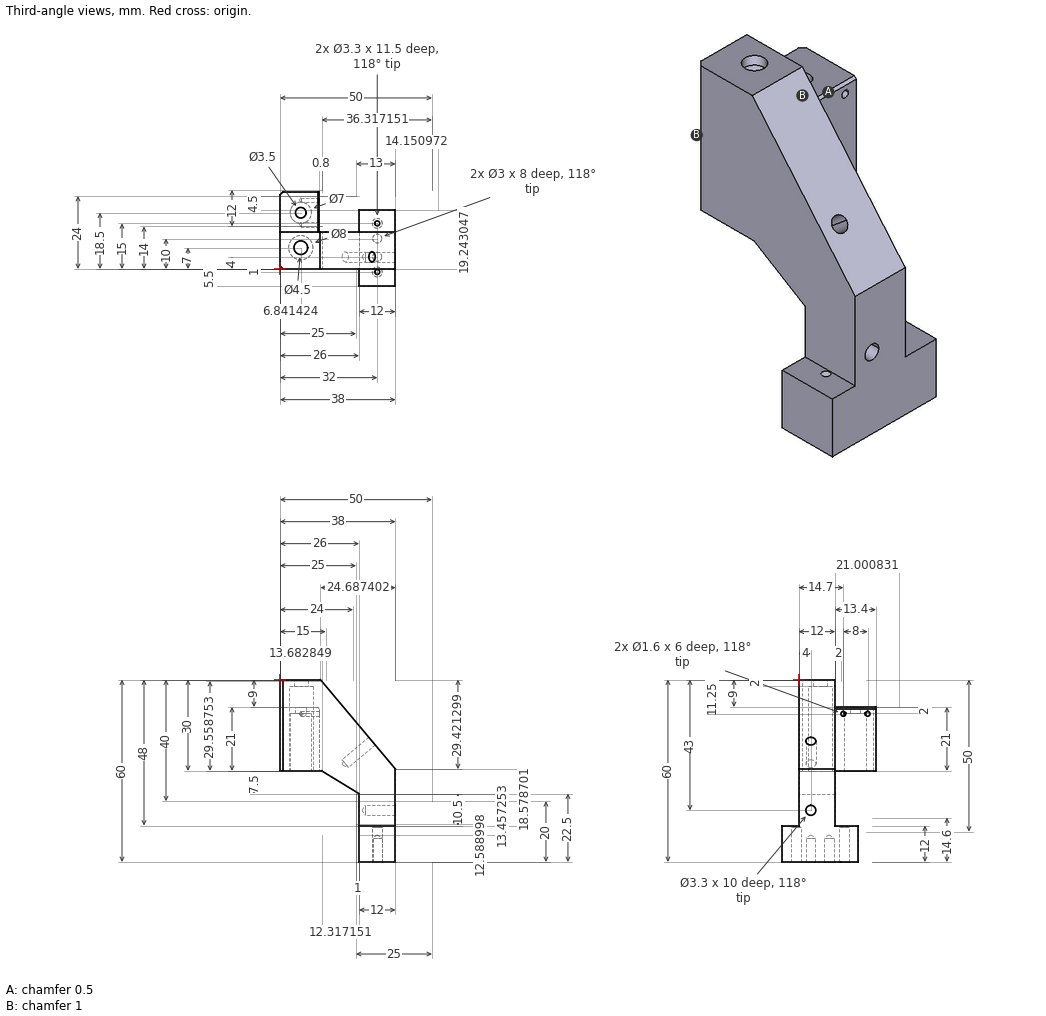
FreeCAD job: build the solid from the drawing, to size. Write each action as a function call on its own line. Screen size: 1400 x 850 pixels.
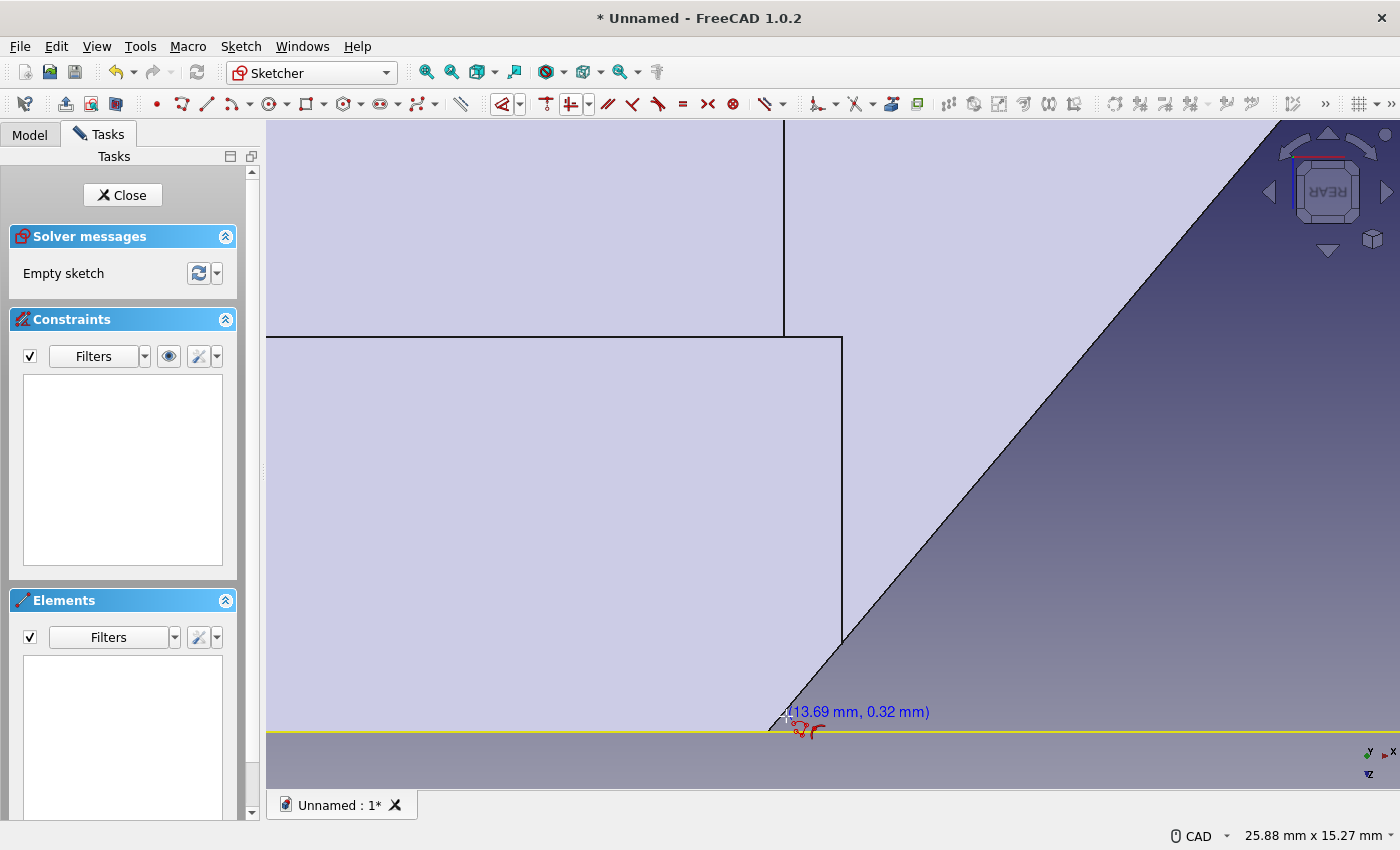
click(784, 712)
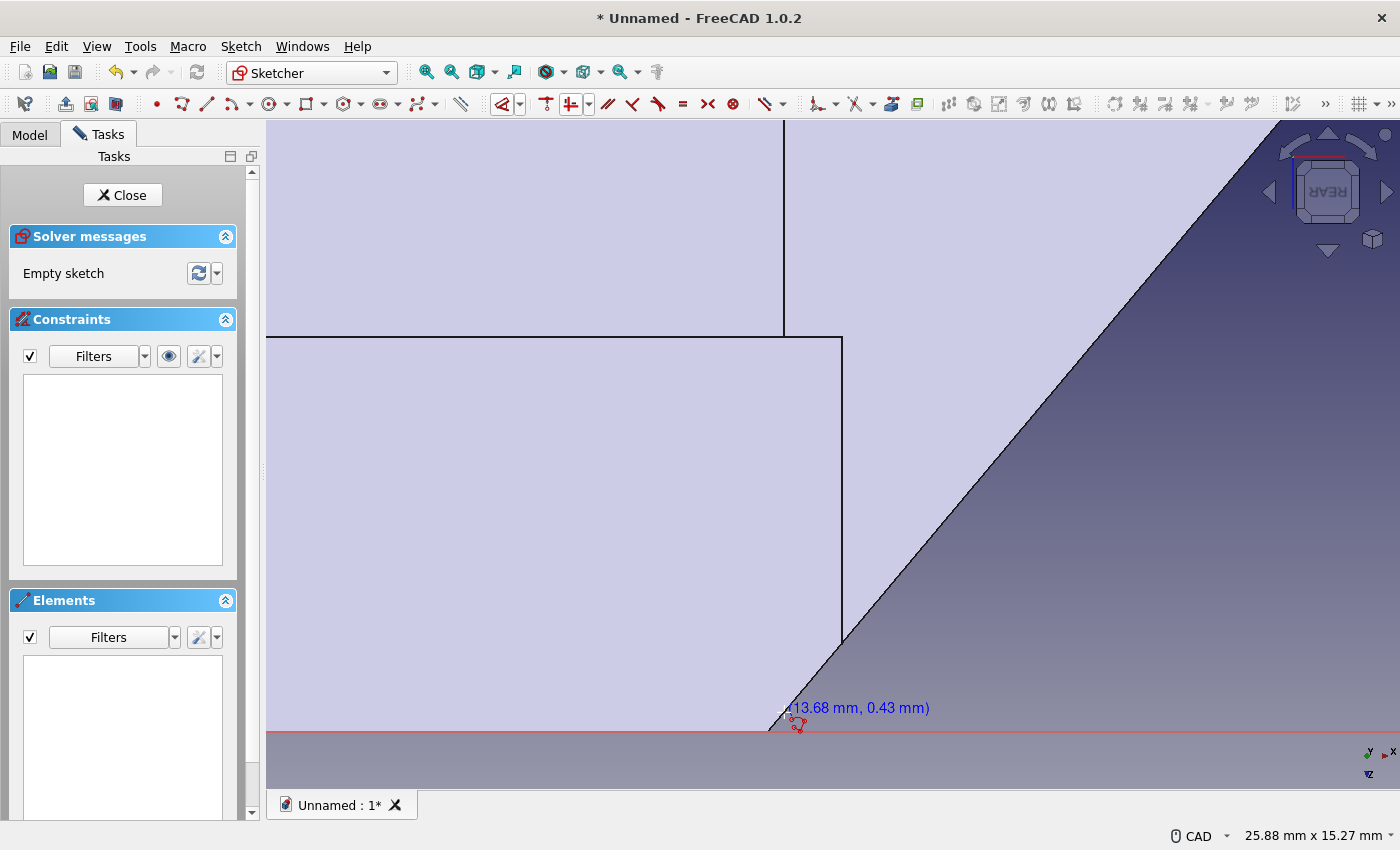
scroll(701, 650, down, 8)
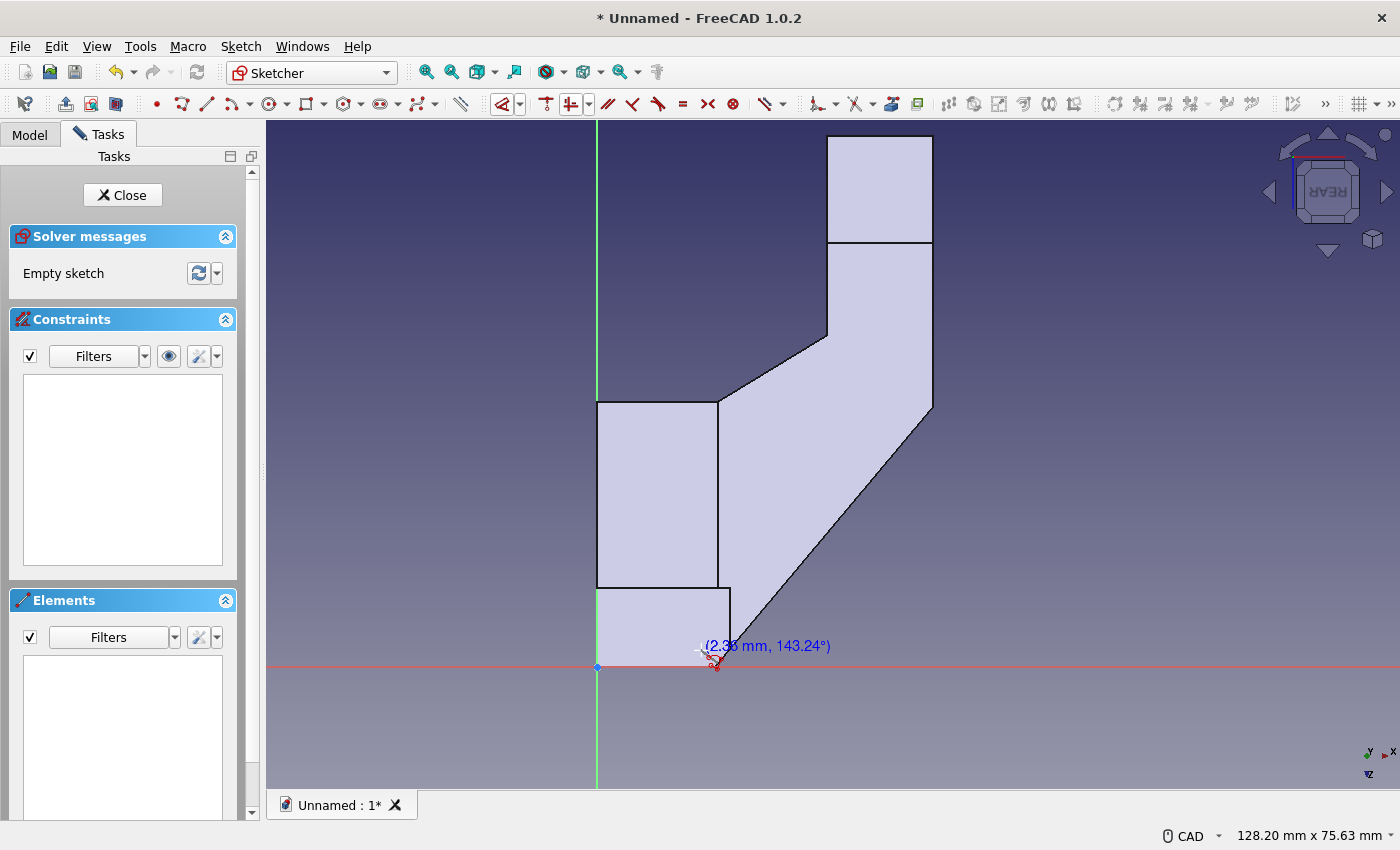
click(933, 407)
click(933, 243)
click(827, 243)
click(827, 335)
click(718, 402)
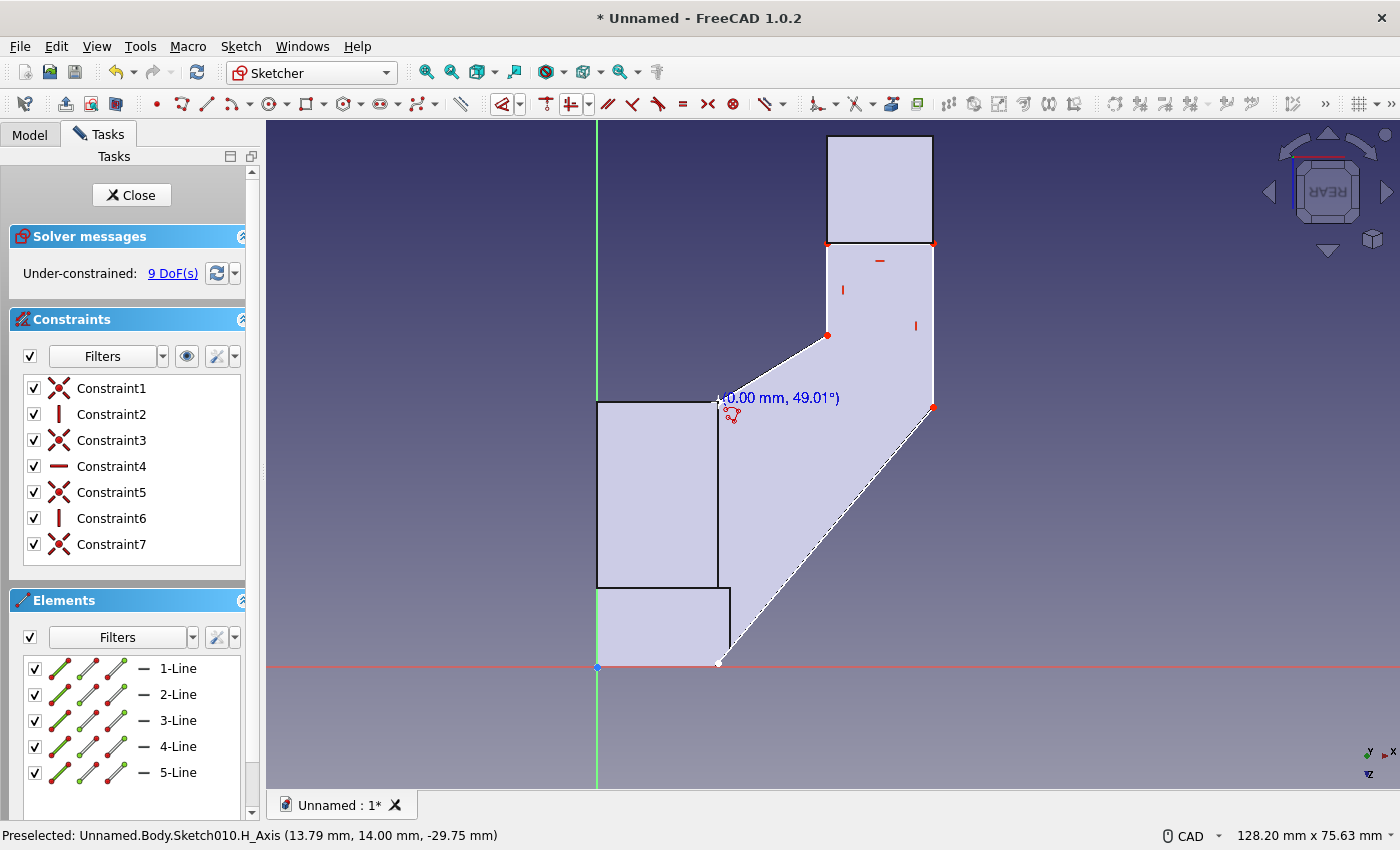
scroll(718, 663, up, 8)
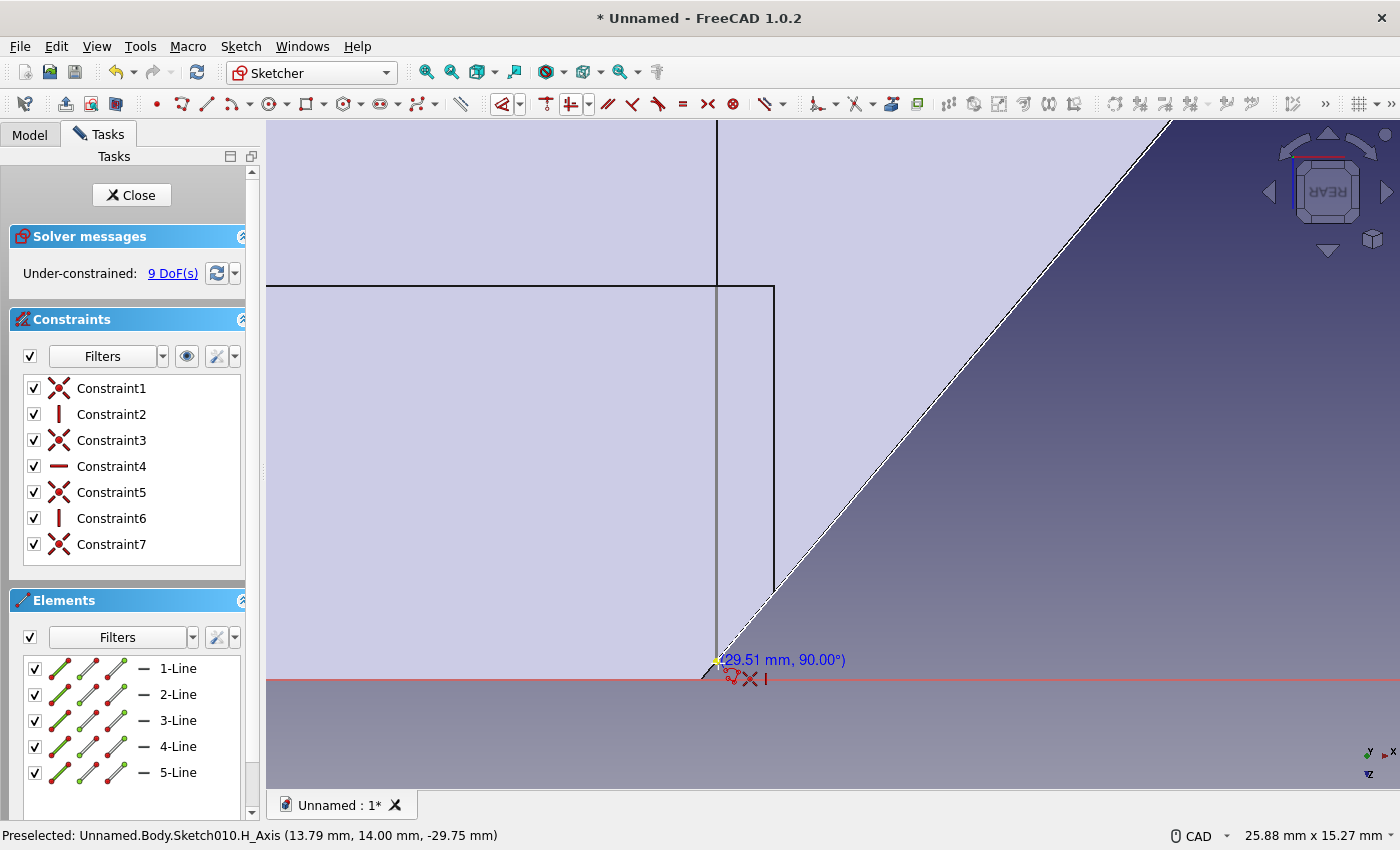
click(717, 662)
key(Escape)
key(Escape)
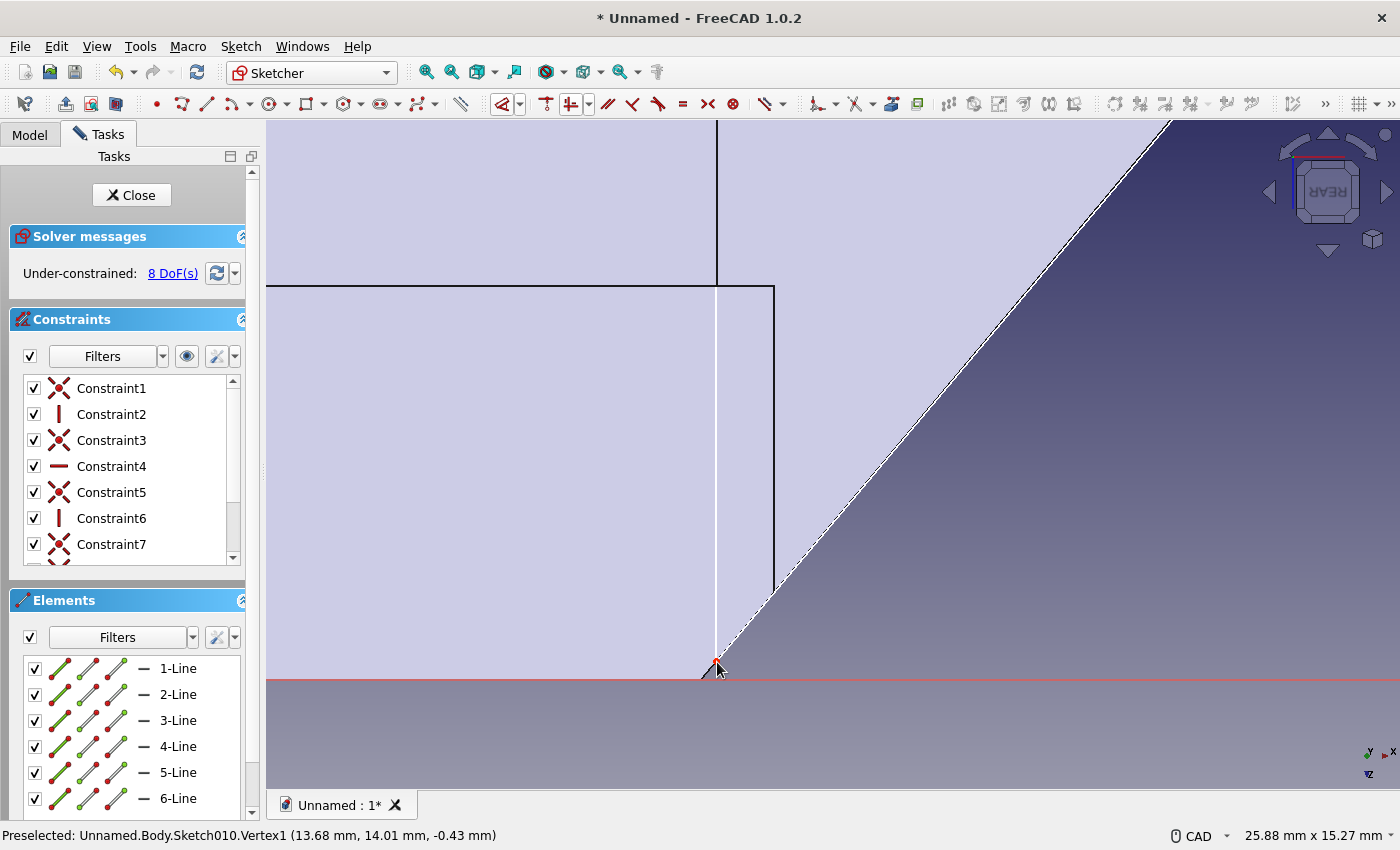
scroll(718, 663, down, 8)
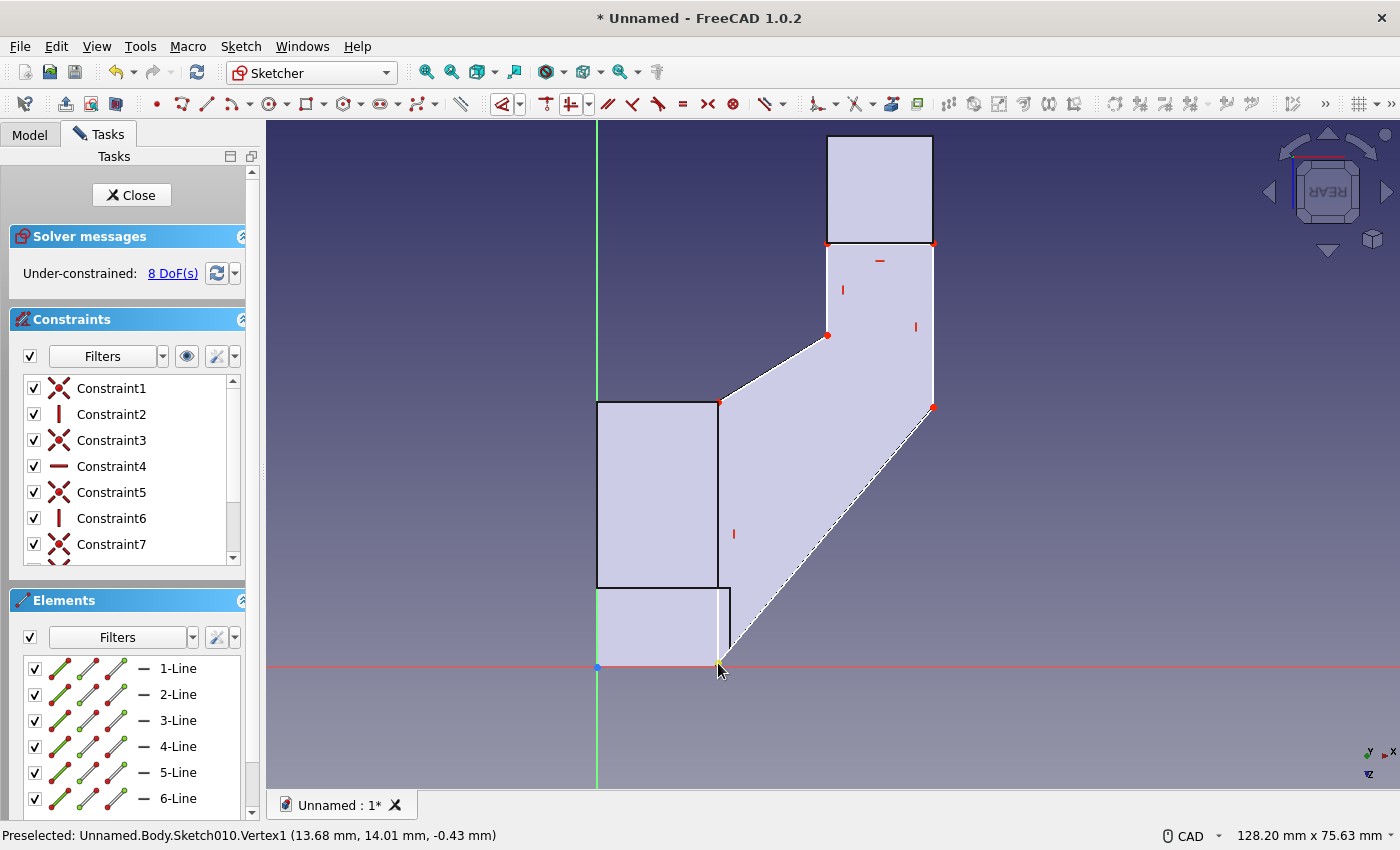
click(901, 244)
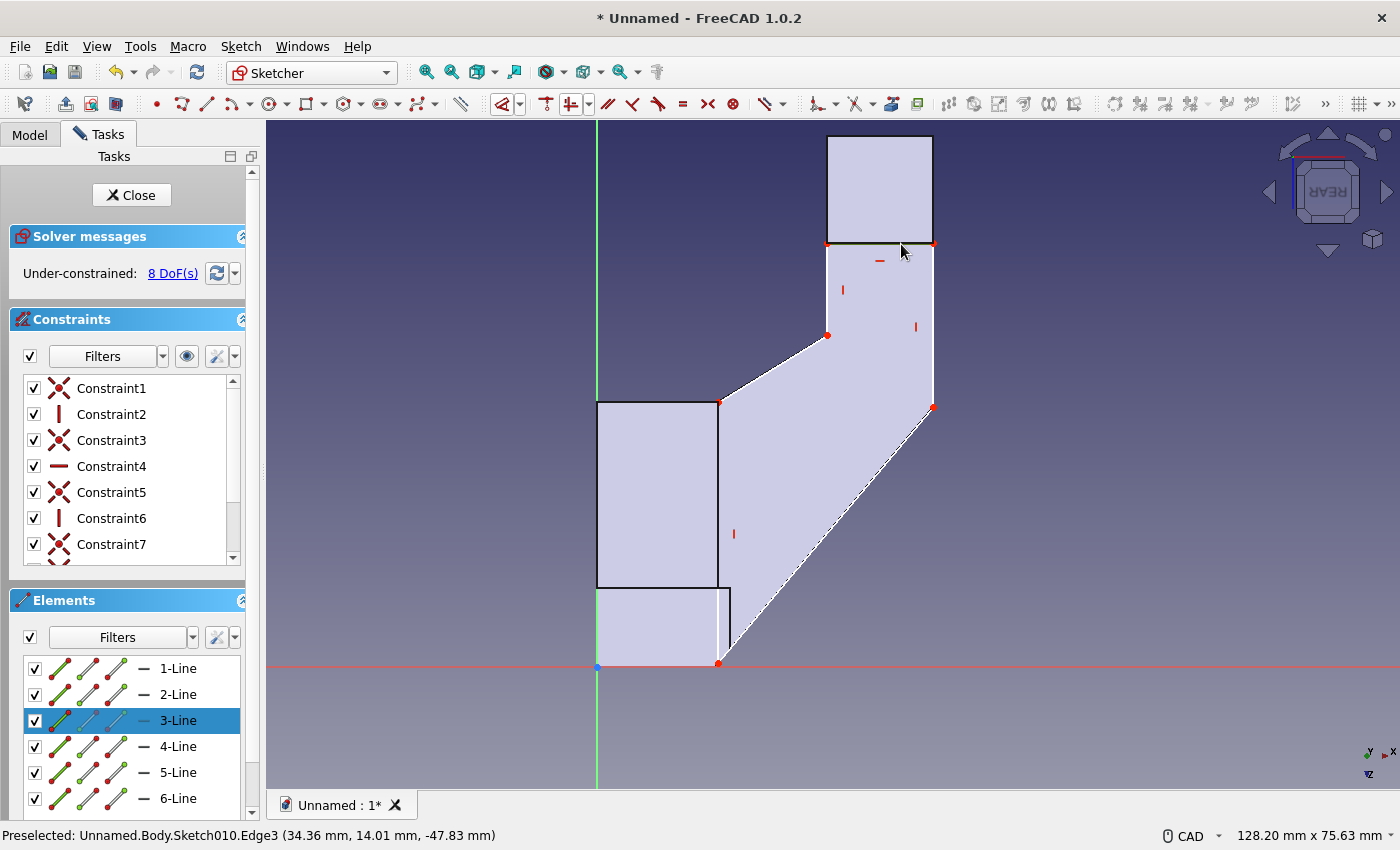
key(l)